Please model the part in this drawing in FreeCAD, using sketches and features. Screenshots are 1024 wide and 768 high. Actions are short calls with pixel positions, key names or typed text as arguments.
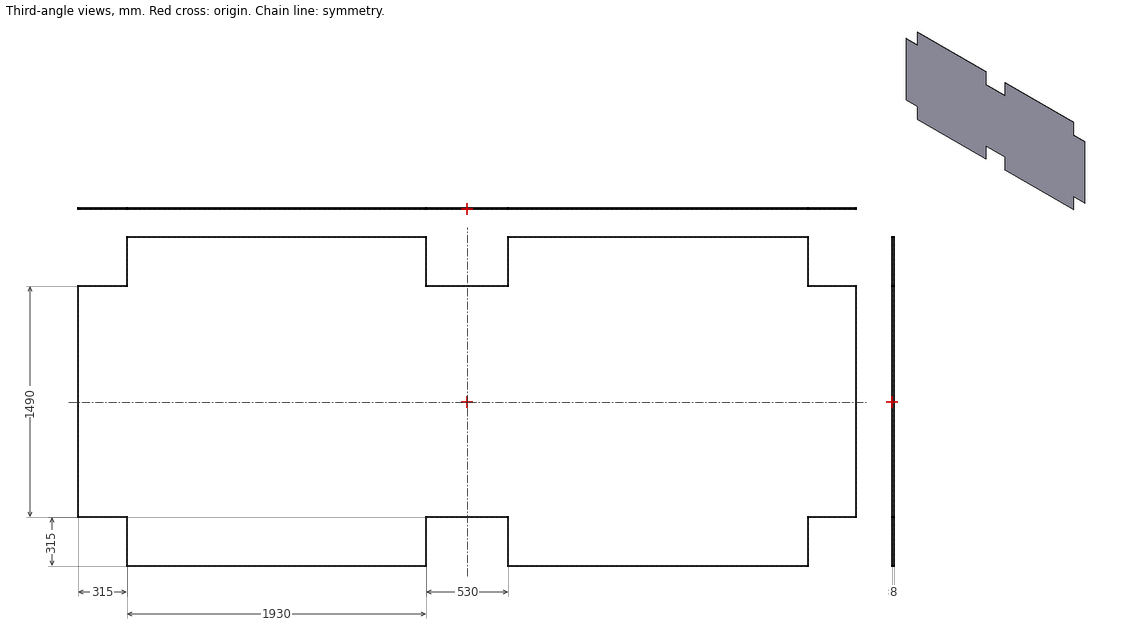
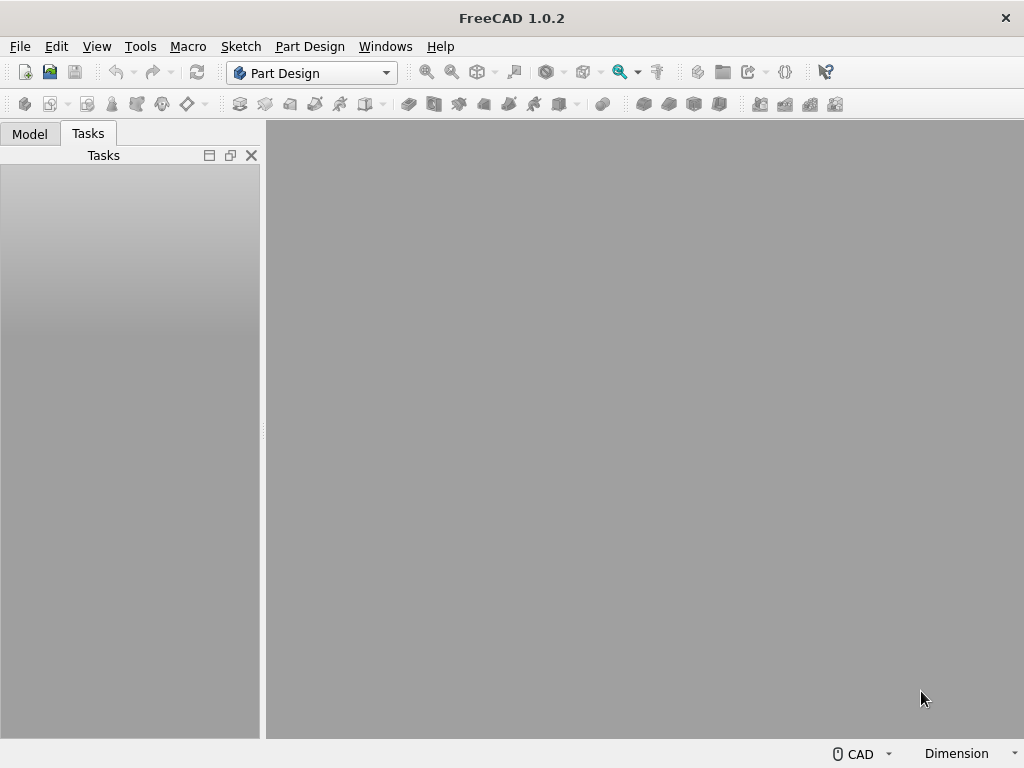
click(25, 72)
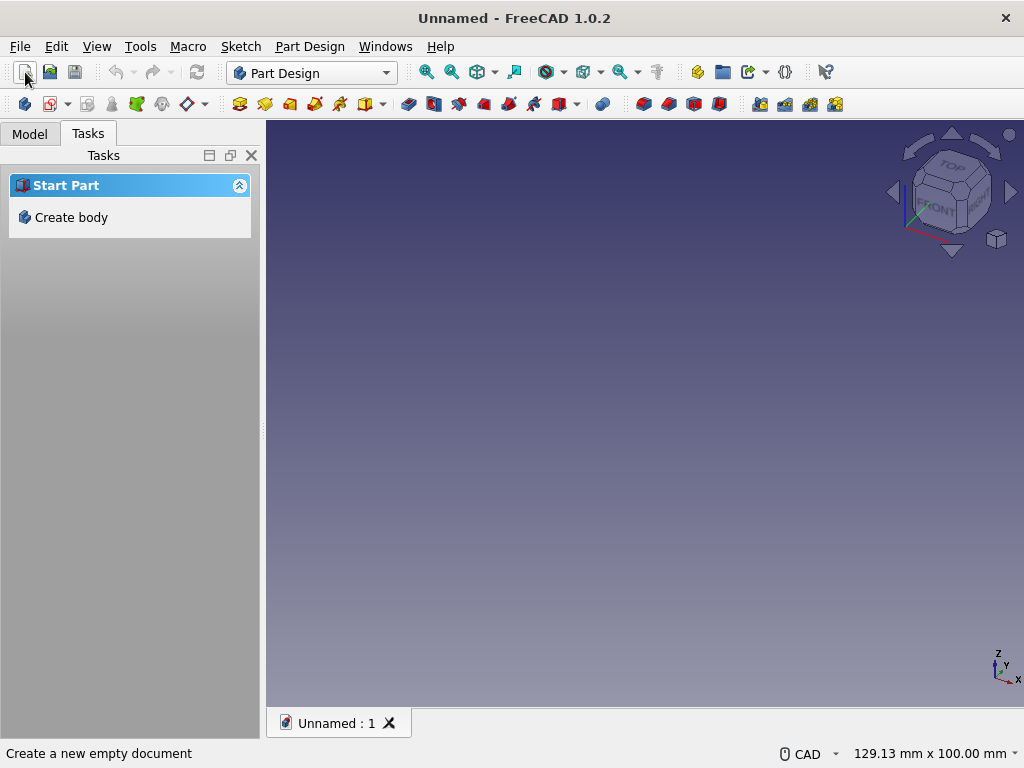
click(50, 104)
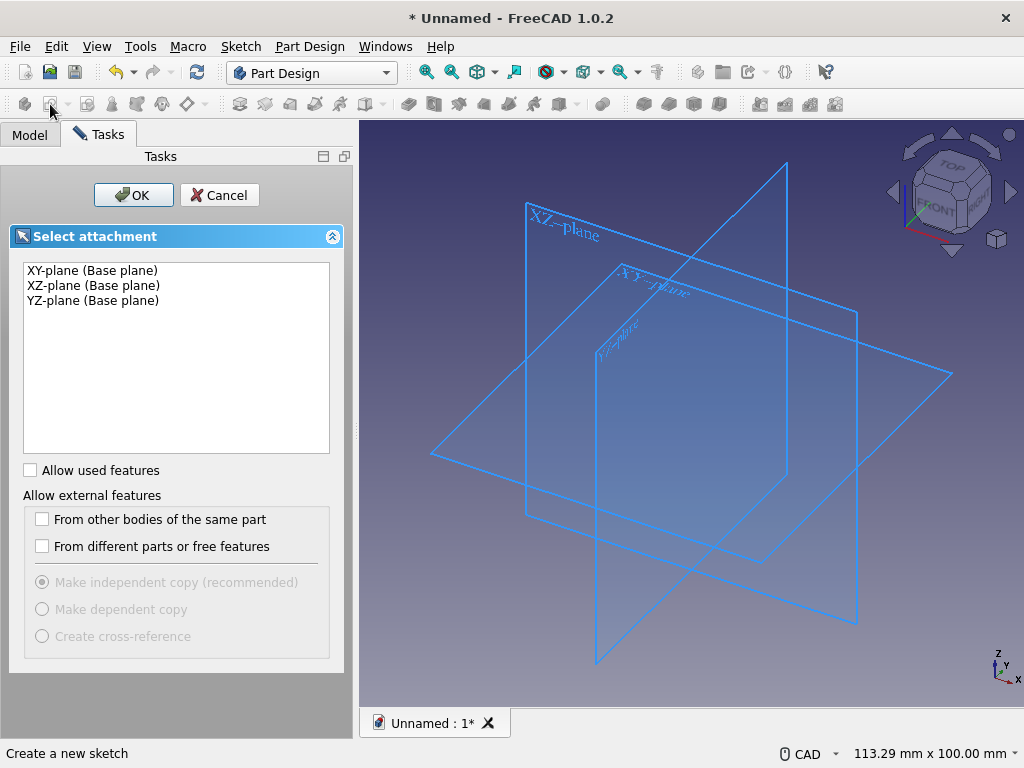
click(84, 286)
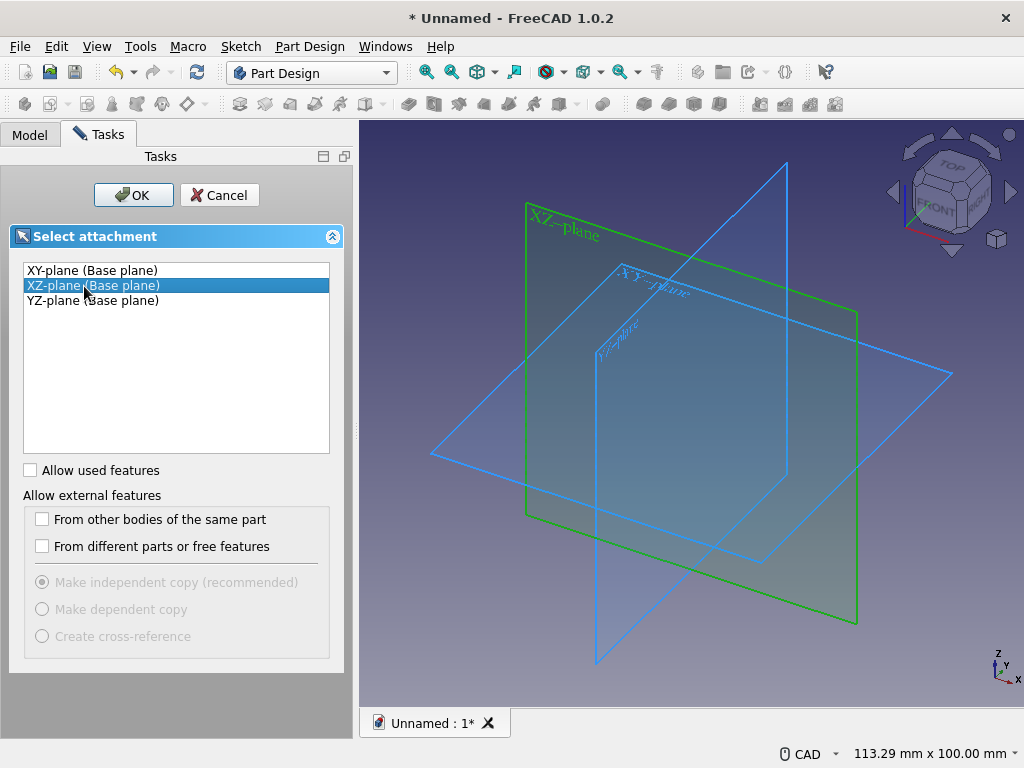
click(134, 195)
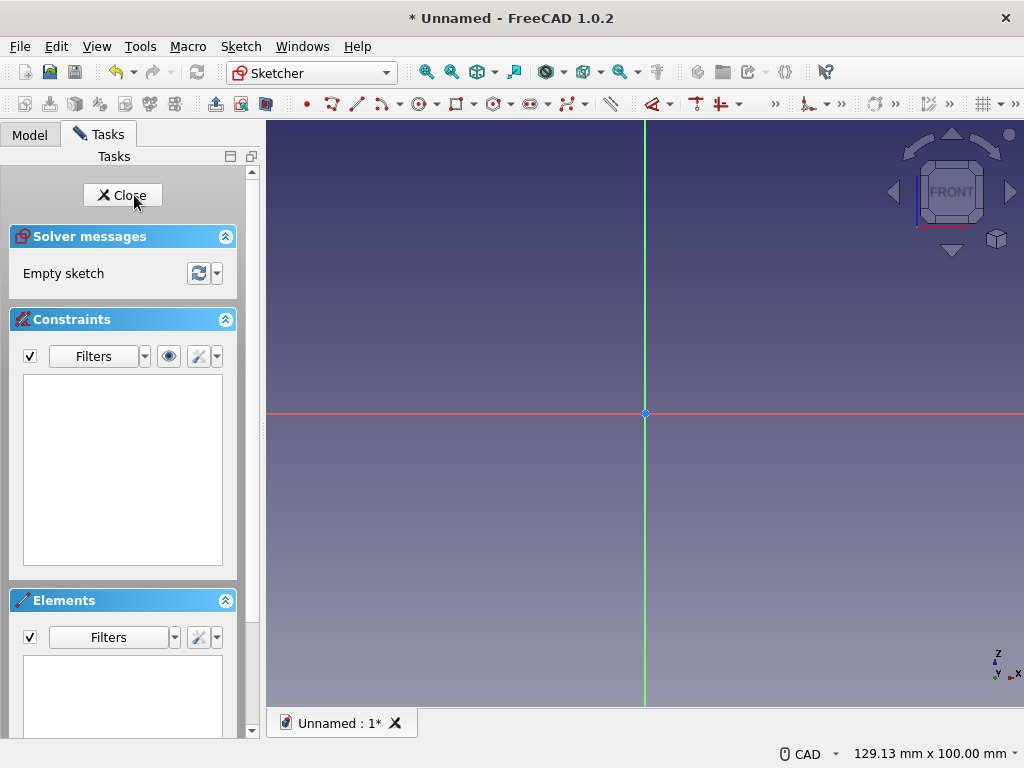
scroll(576, 414, down, 15)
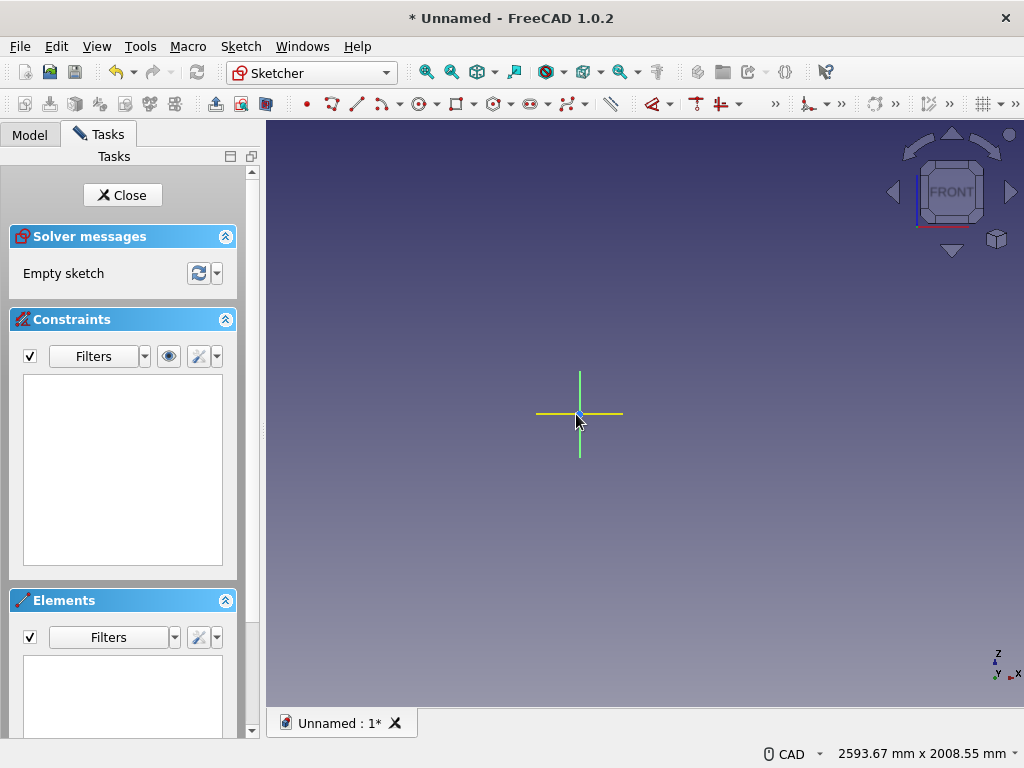
scroll(575, 413, down, 7)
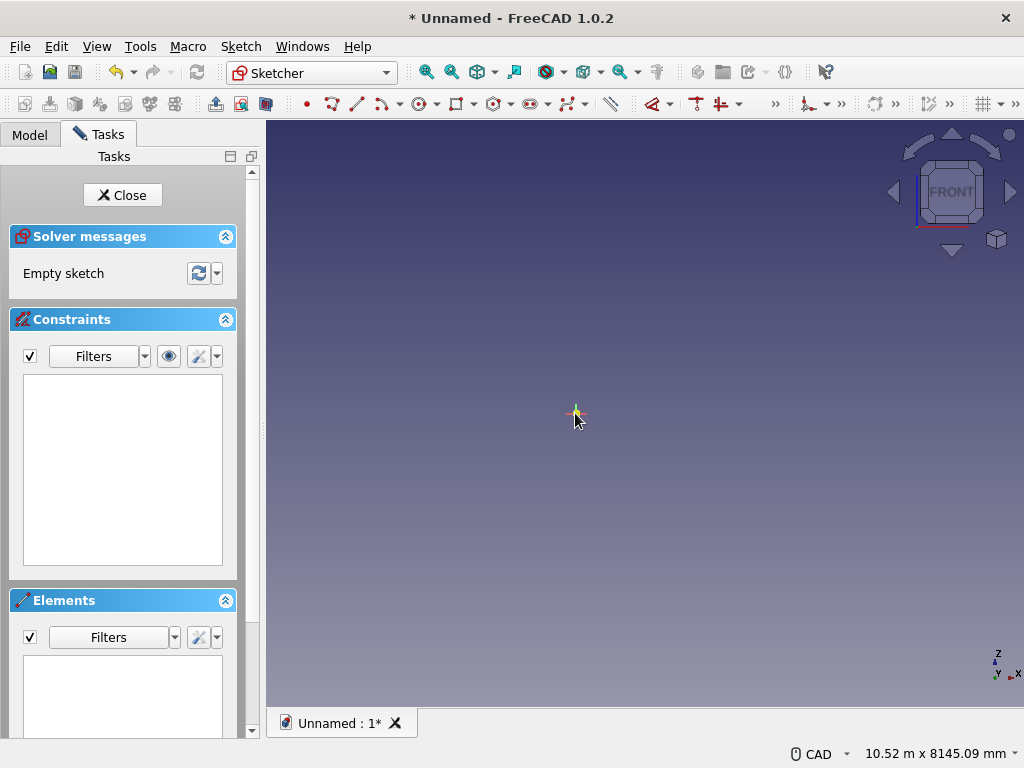
click(332, 104)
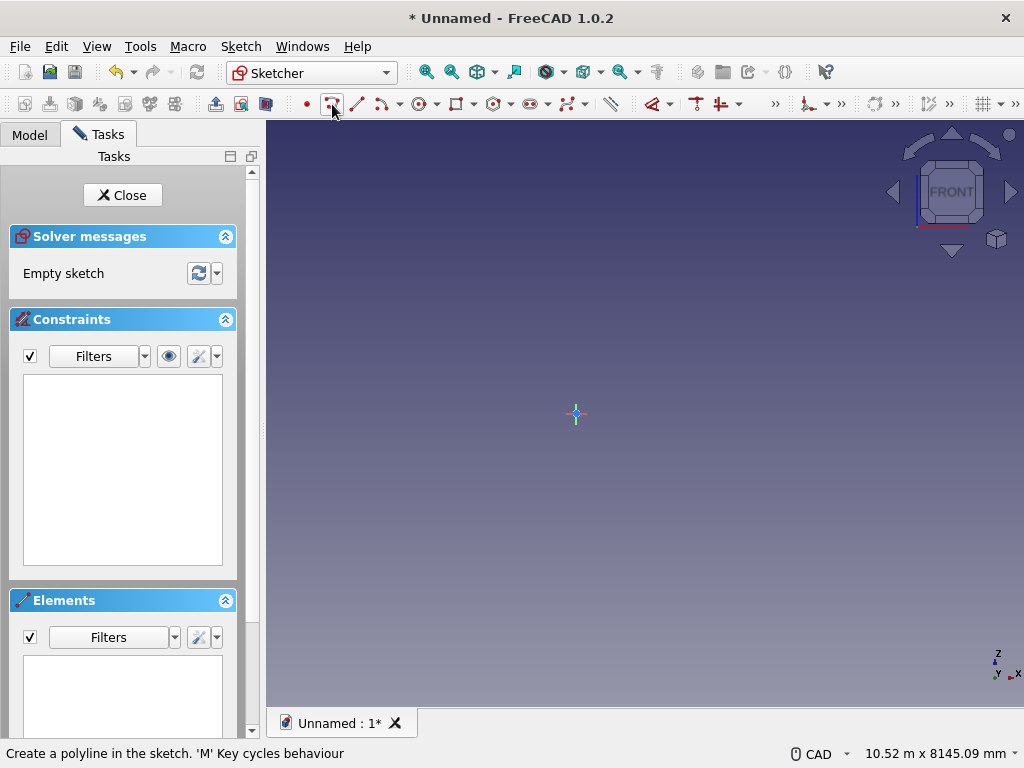
click(596, 467)
click(557, 467)
click(557, 490)
click(418, 490)
click(418, 467)
click(396, 467)
click(396, 360)
click(418, 360)
click(418, 337)
click(557, 337)
click(557, 360)
click(596, 360)
click(596, 337)
click(735, 337)
click(735, 360)
click(757, 360)
click(757, 467)
click(735, 467)
click(735, 490)
click(596, 490)
click(596, 468)
key(Escape)
key(Escape)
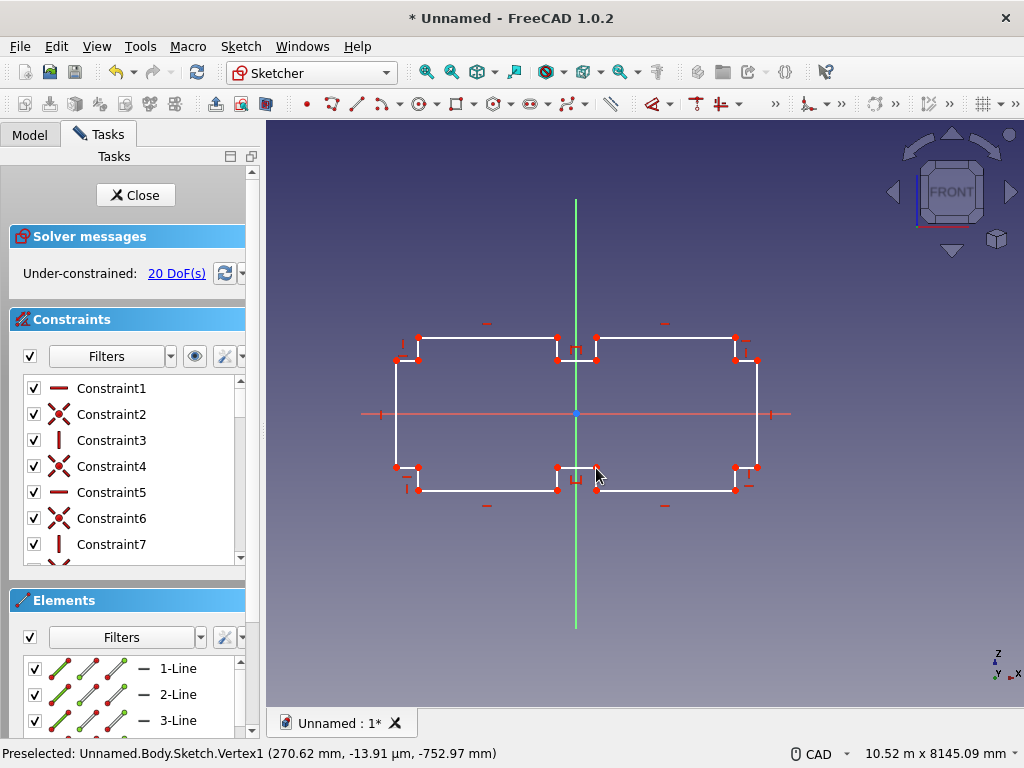
click(418, 468)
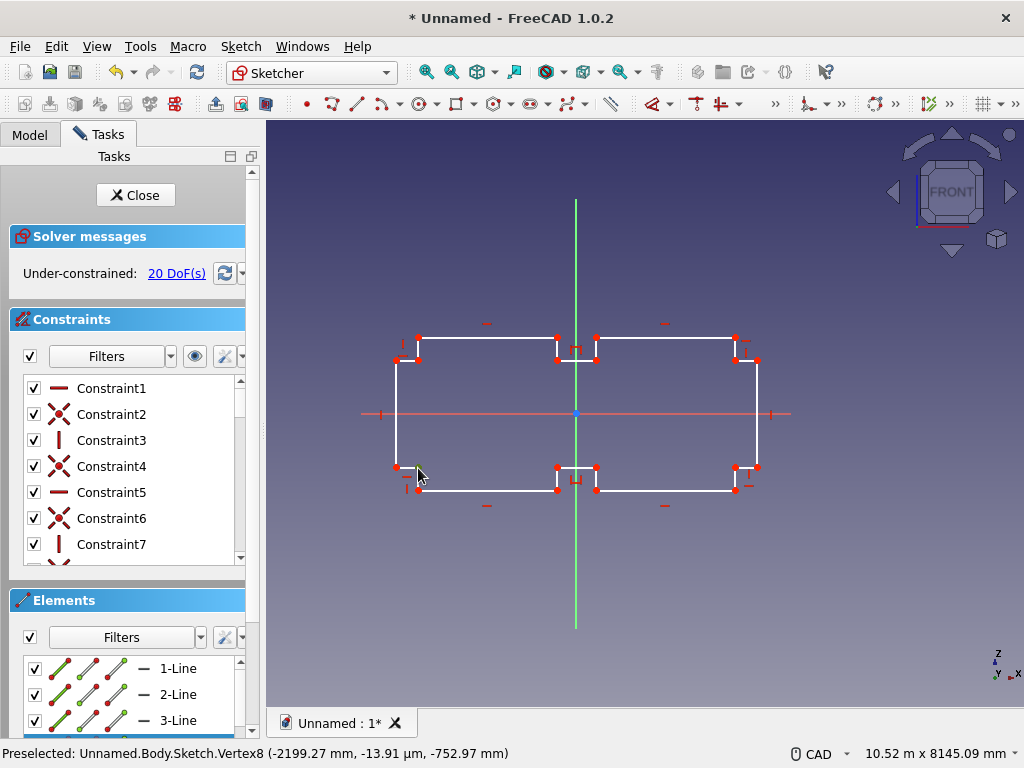
click(418, 361)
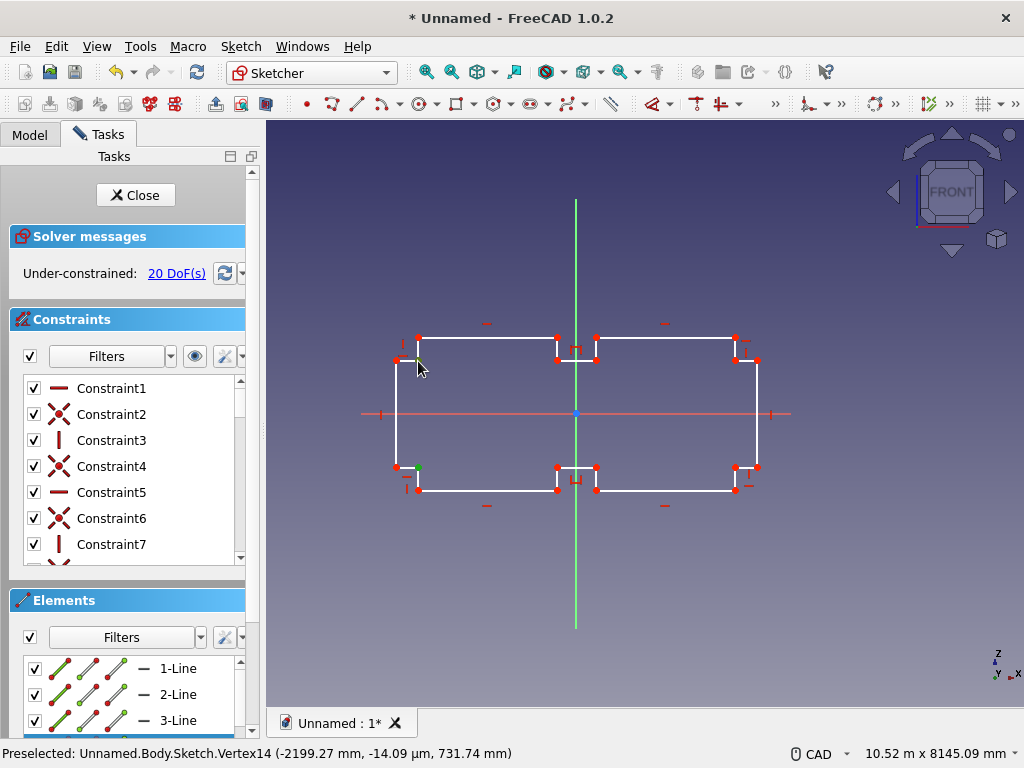
click(455, 414)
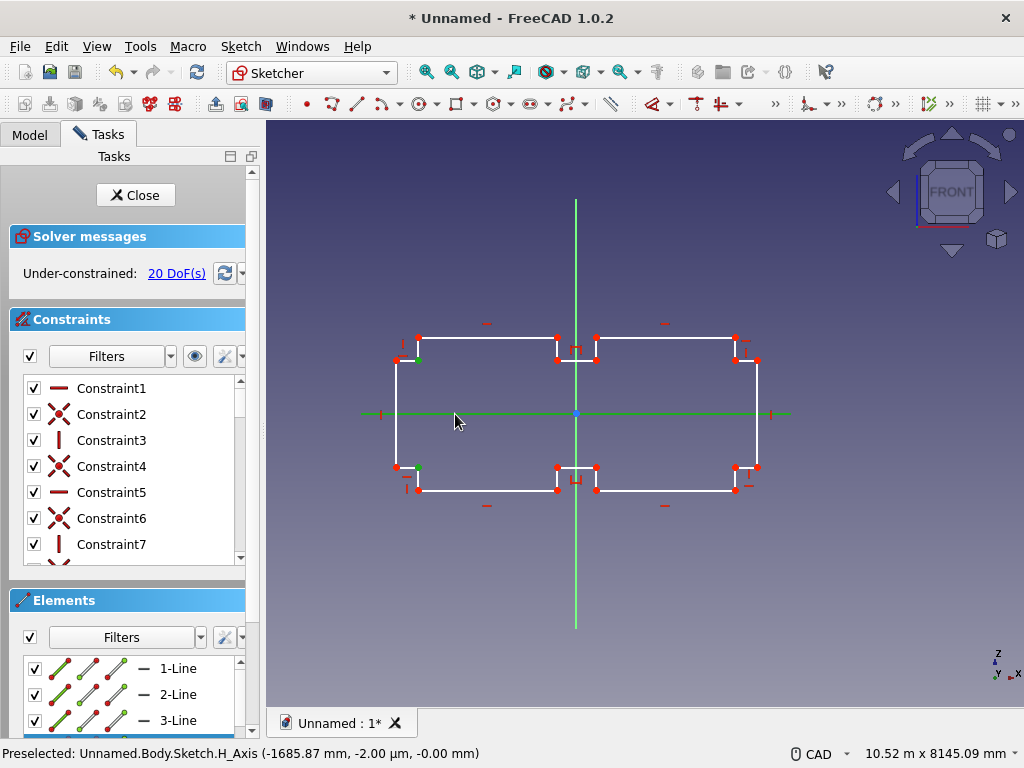
key(s)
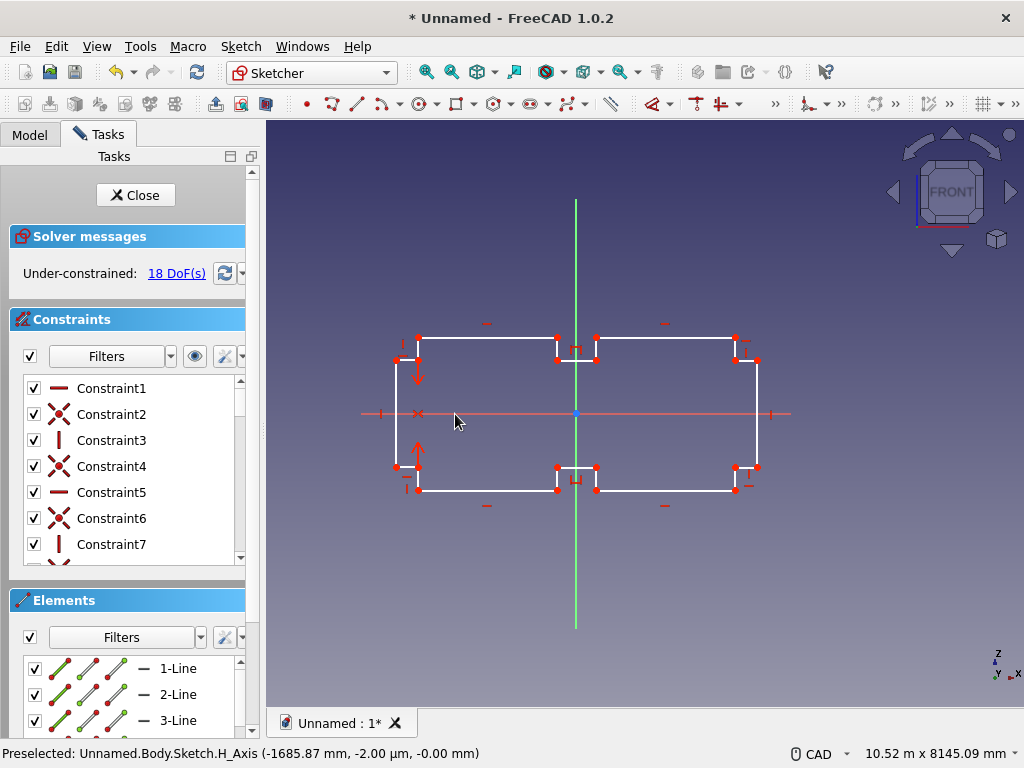
click(557, 491)